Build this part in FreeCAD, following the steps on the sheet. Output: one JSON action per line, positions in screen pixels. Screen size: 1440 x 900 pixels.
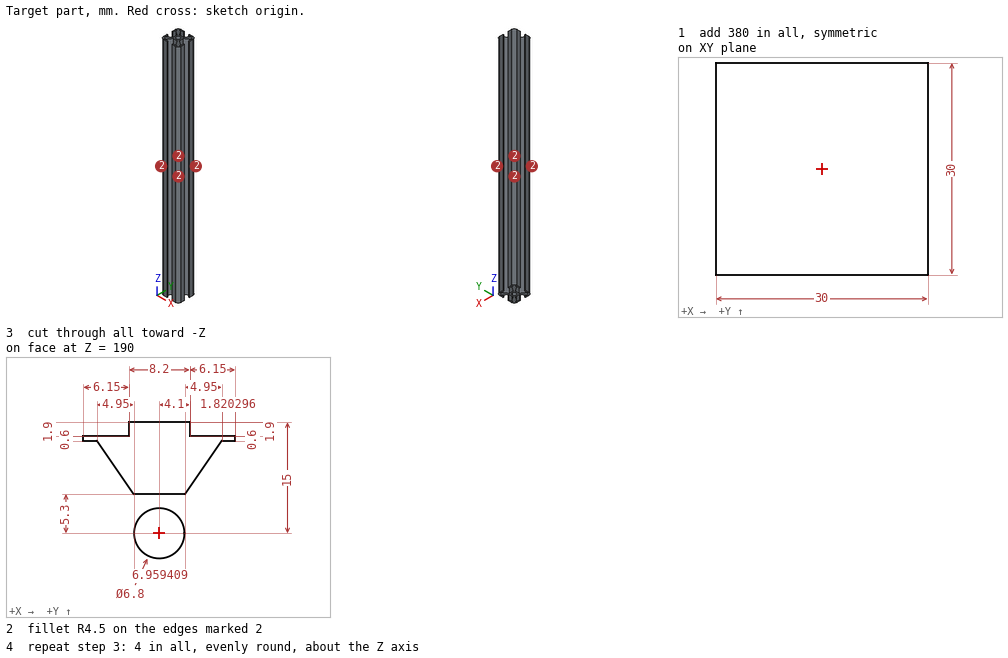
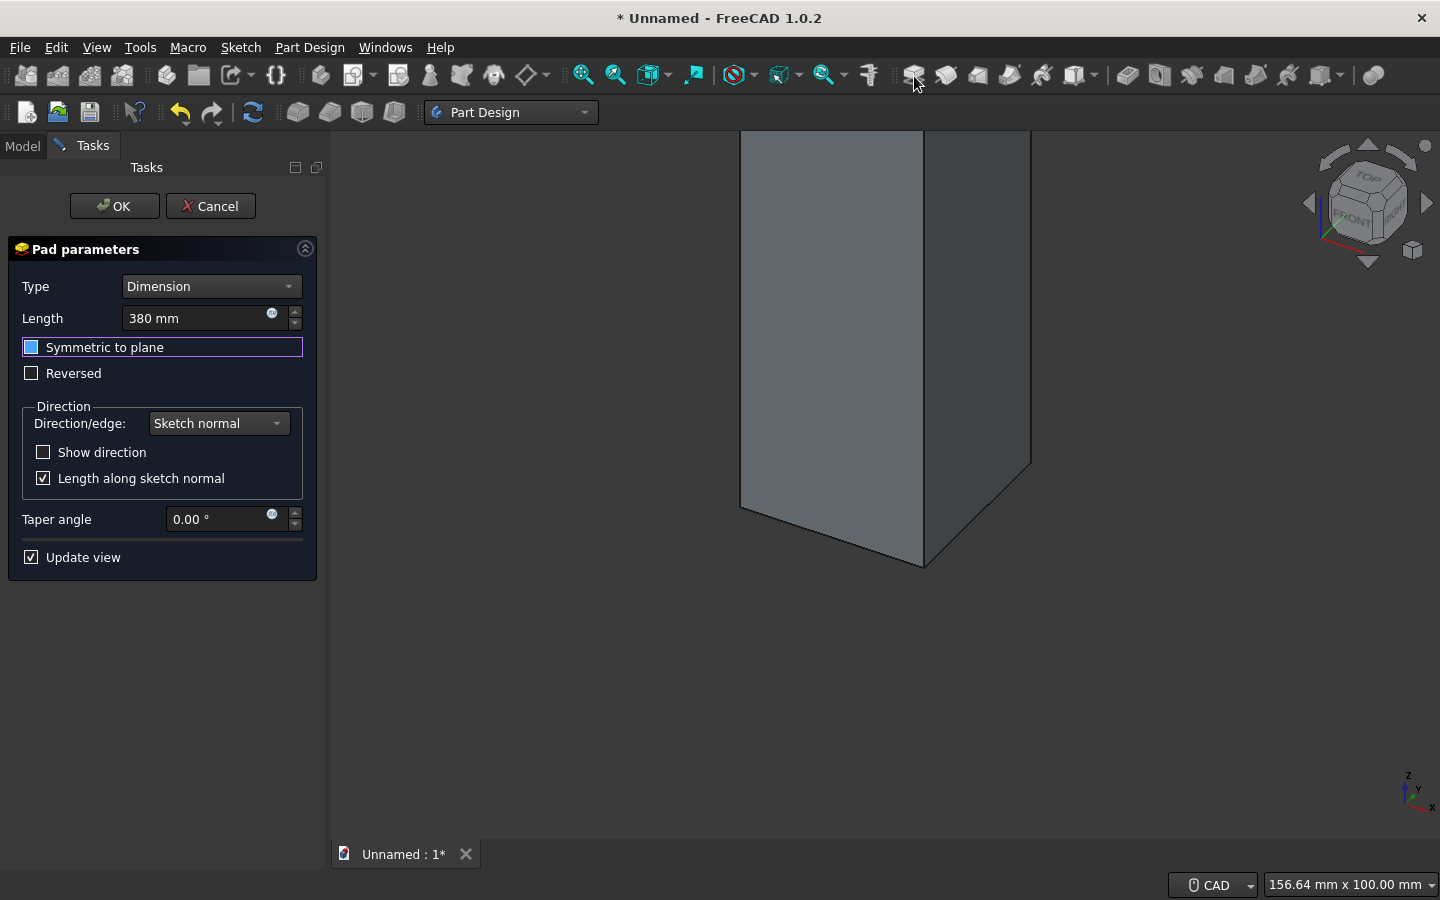
{"action": "left_click", "coordinate": [30, 347]}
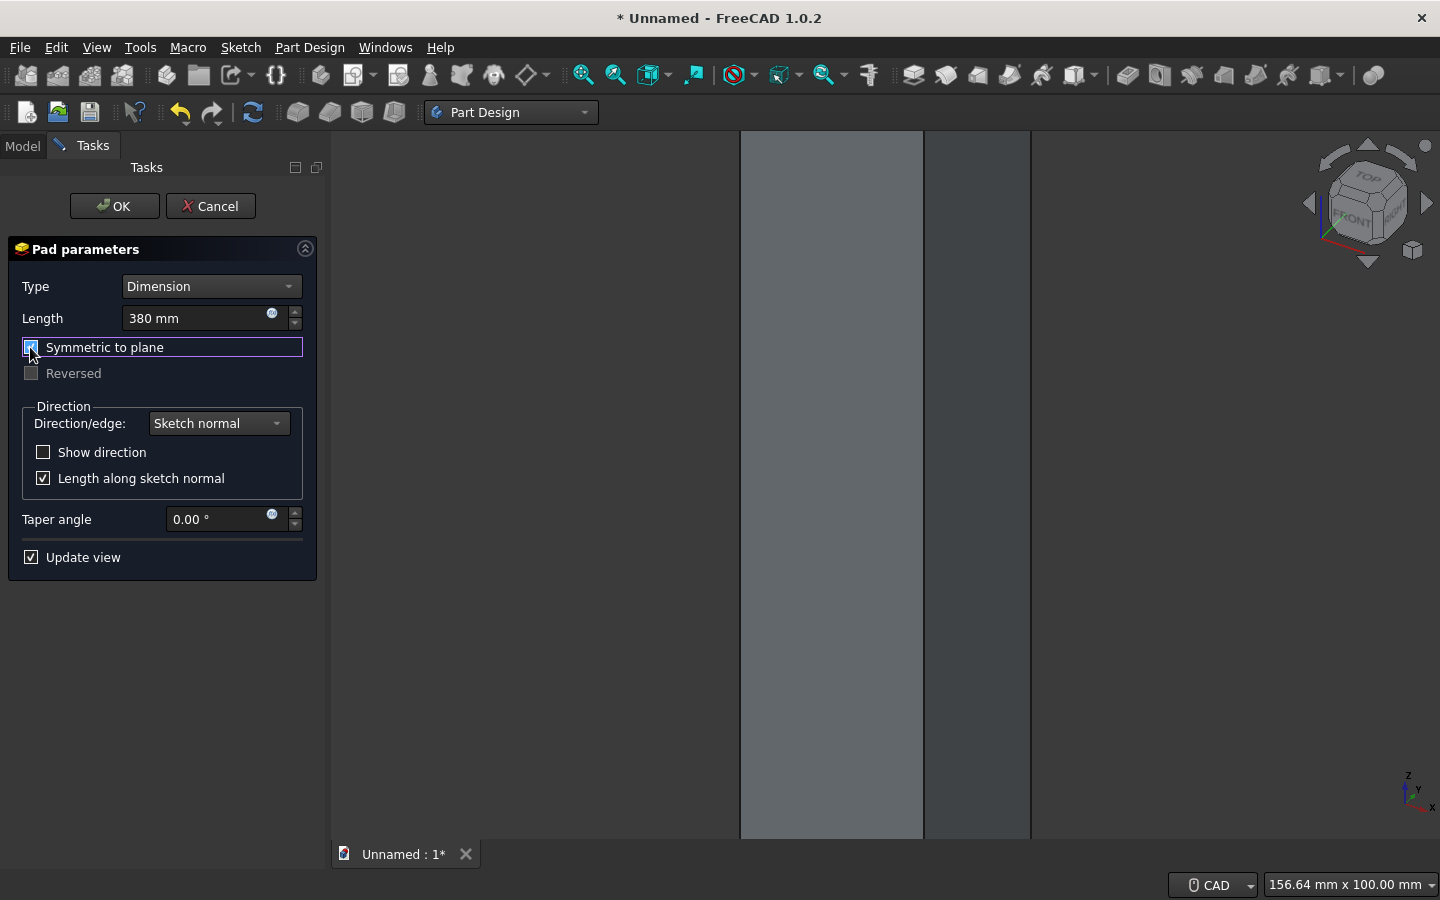
{"action": "left_click", "coordinate": [115, 206]}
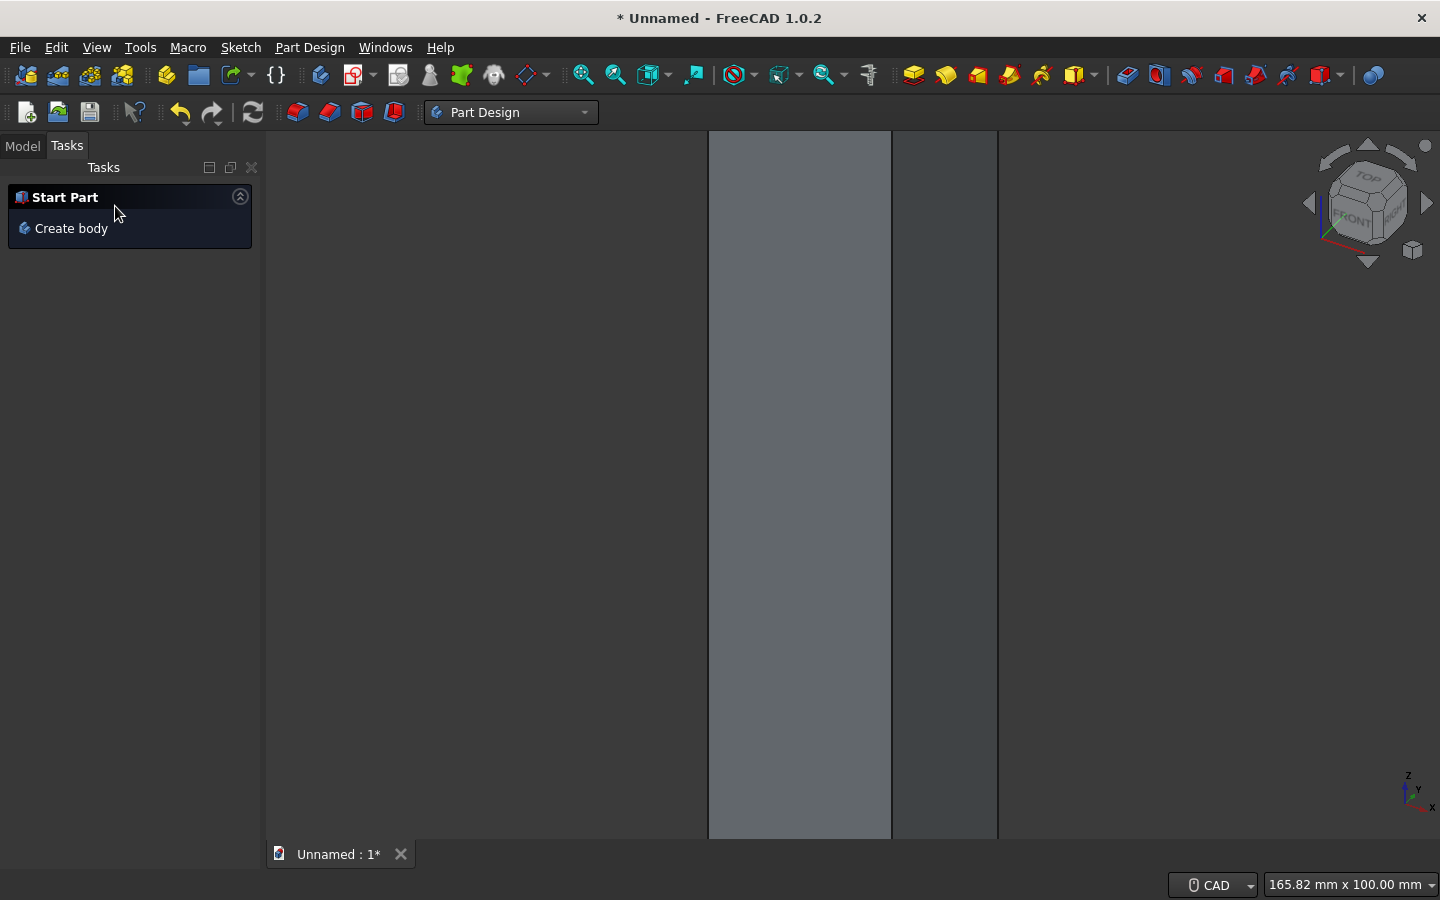
{"action": "left_click", "coordinate": [584, 76]}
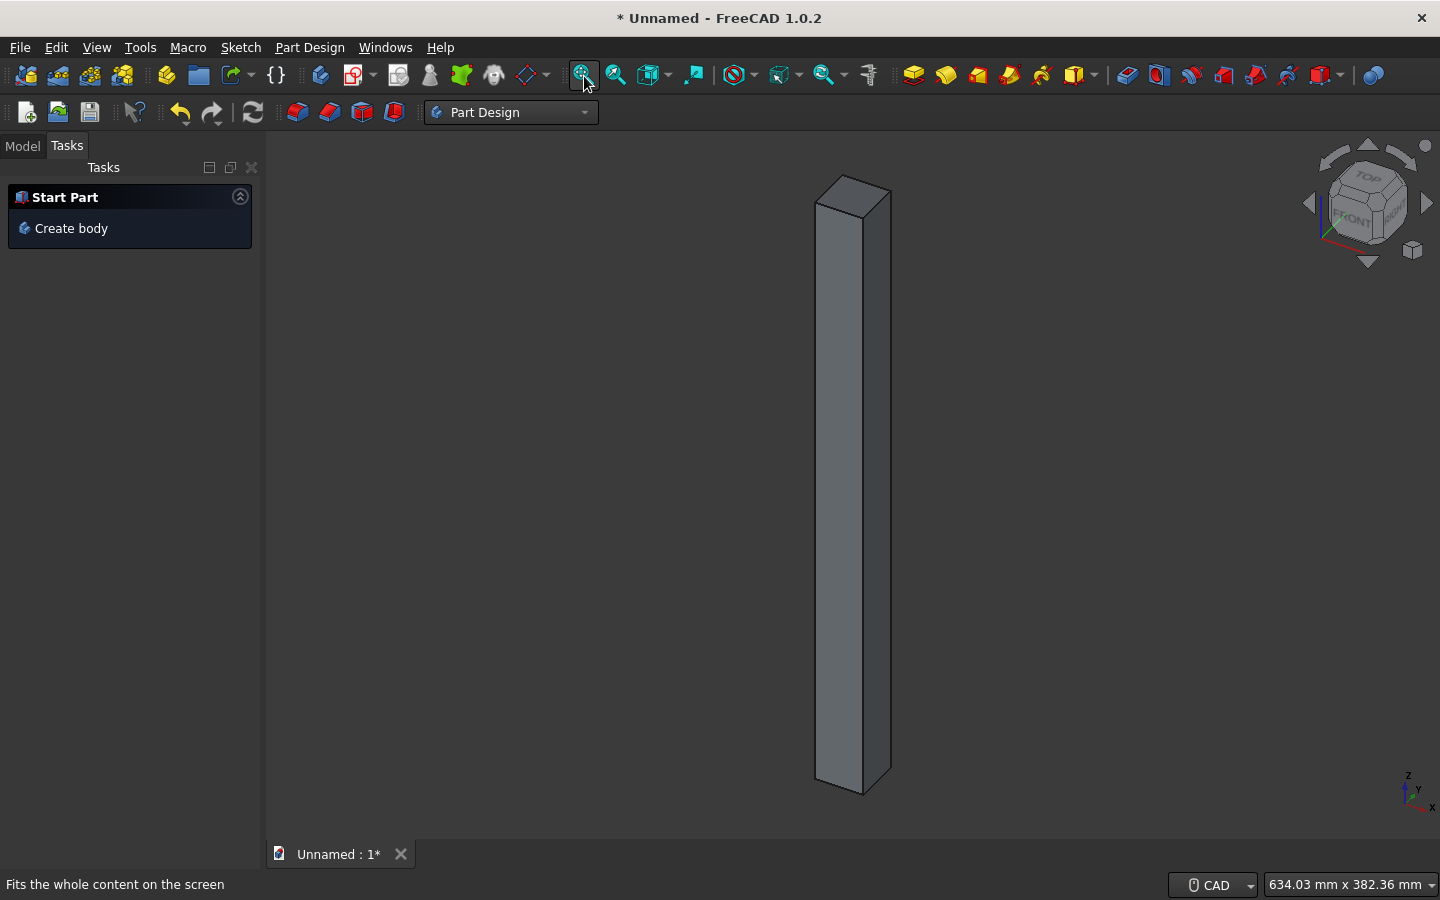
{"action": "left_click", "coordinate": [863, 506]}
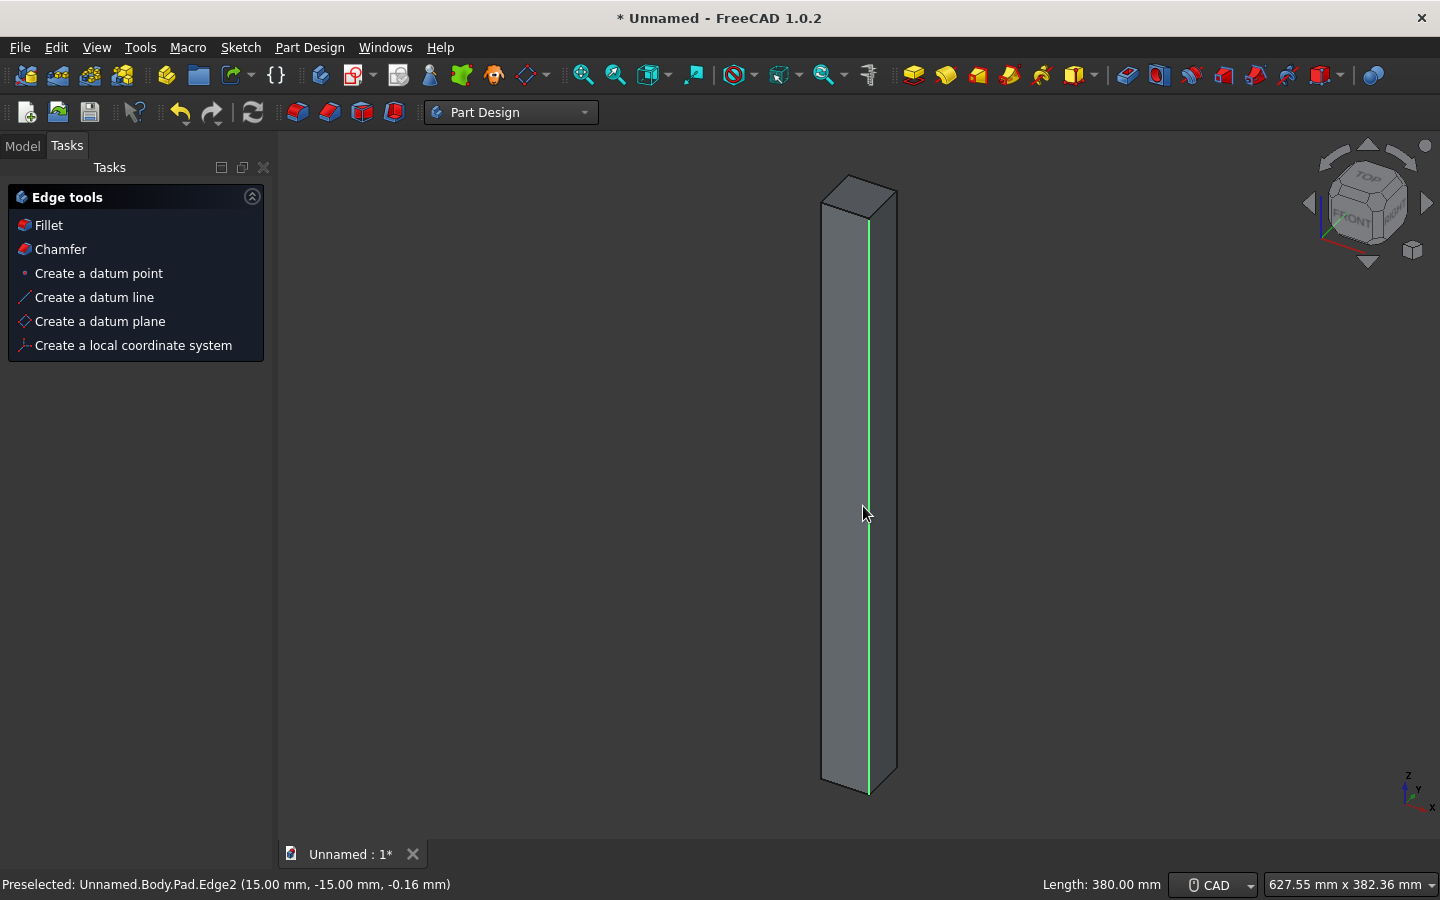
{"action": "key", "text": "0"}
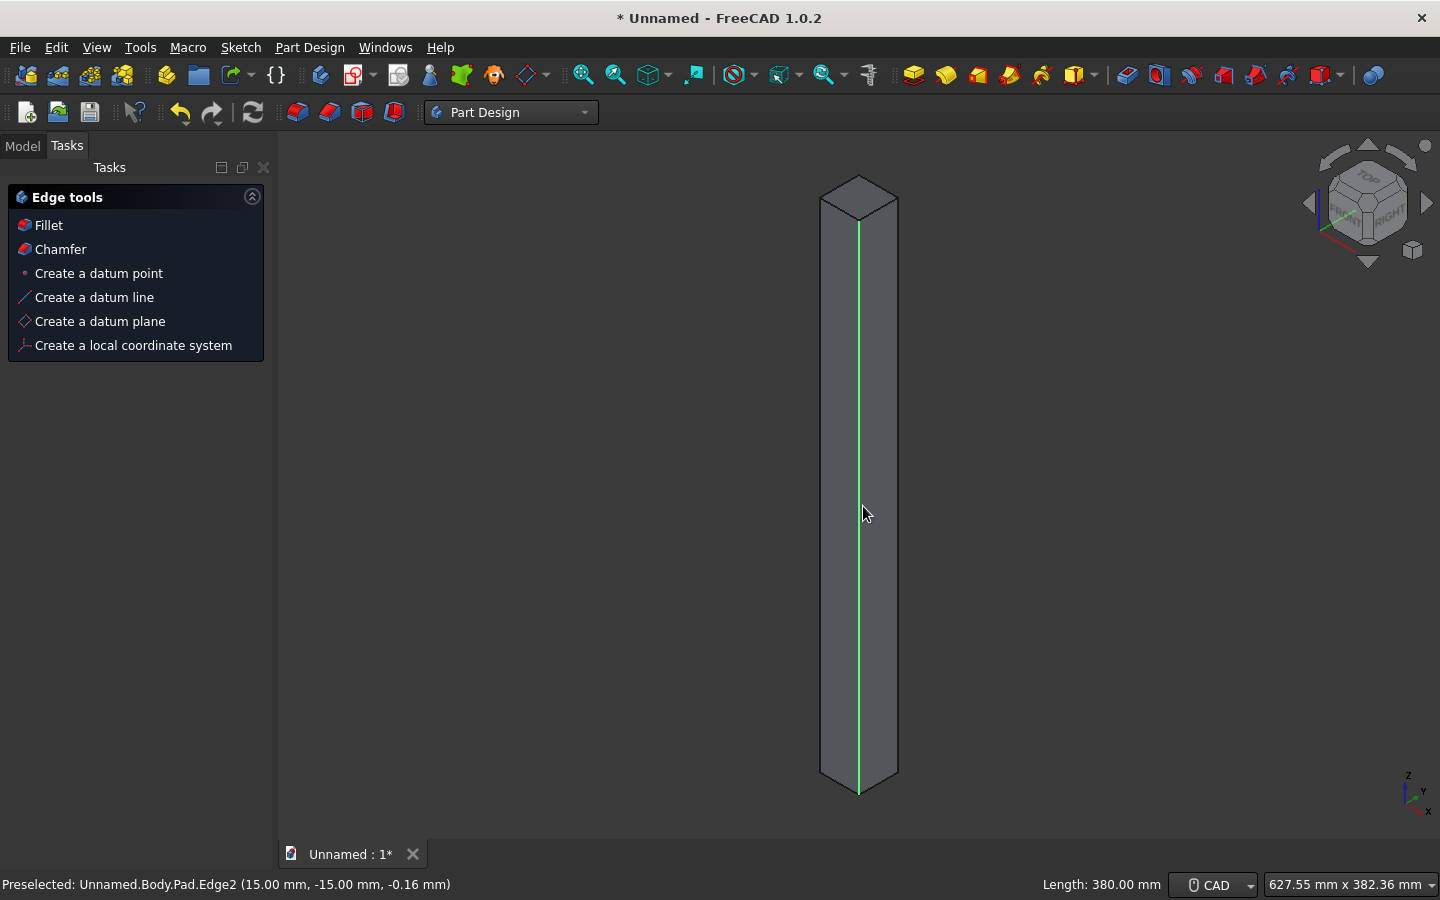
{"action": "key", "text": "2"}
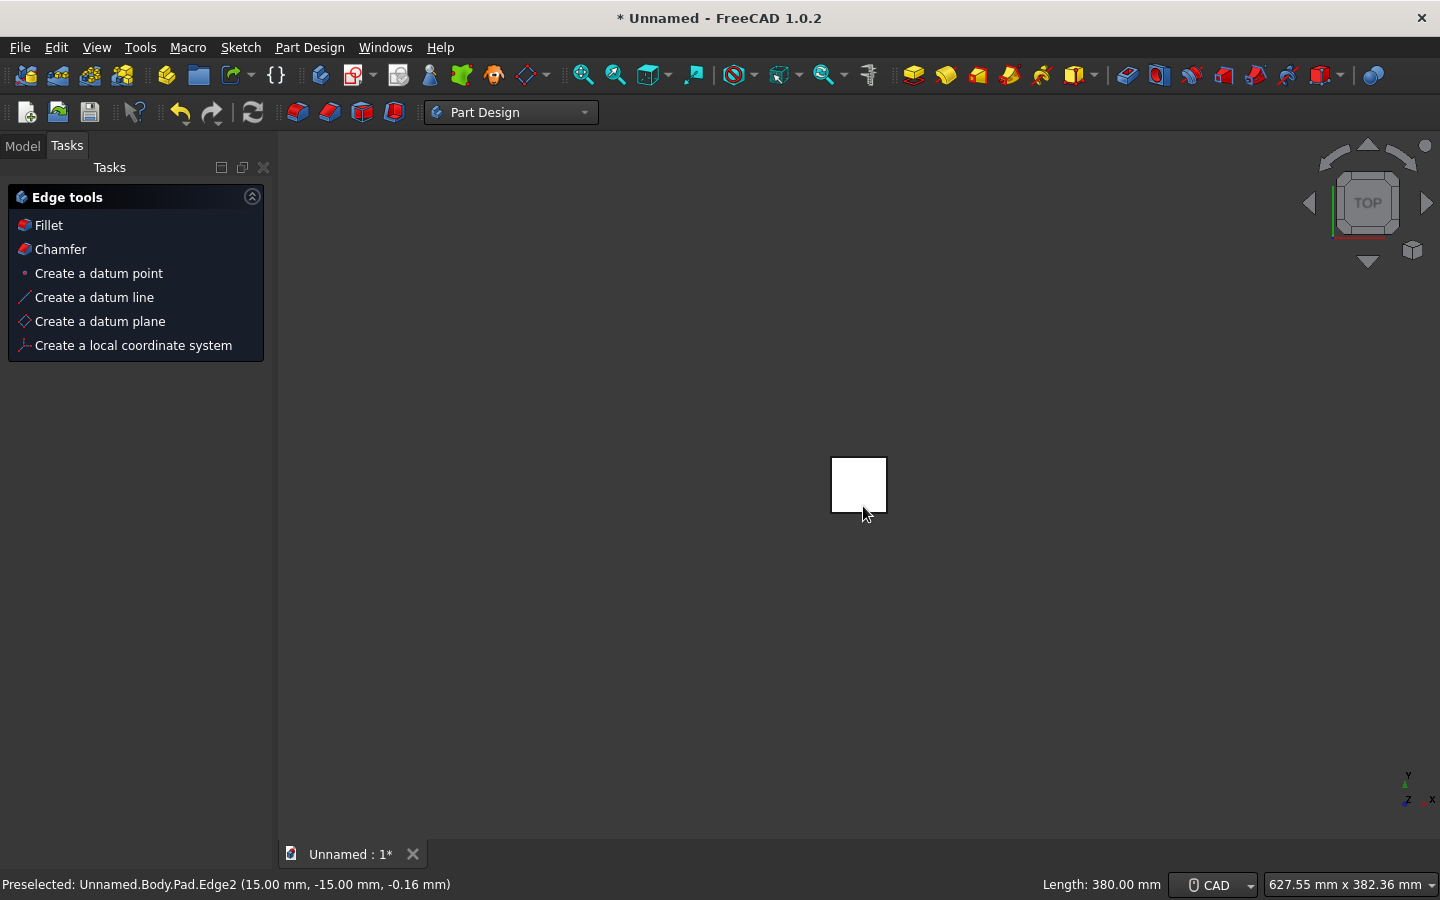
{"action": "left_click", "coordinate": [584, 76]}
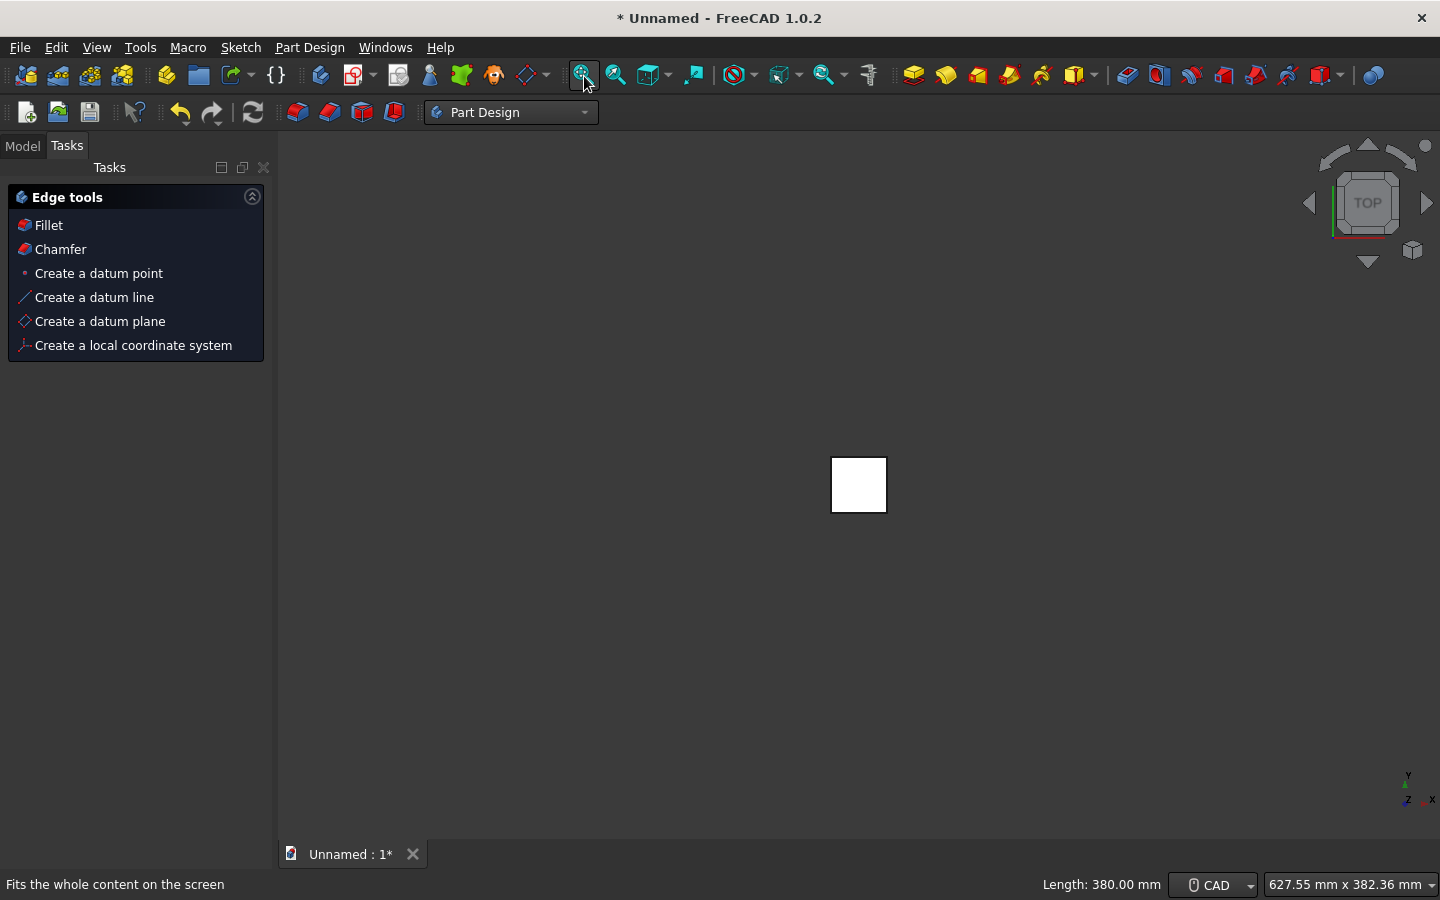
{"action": "key", "text": "1"}